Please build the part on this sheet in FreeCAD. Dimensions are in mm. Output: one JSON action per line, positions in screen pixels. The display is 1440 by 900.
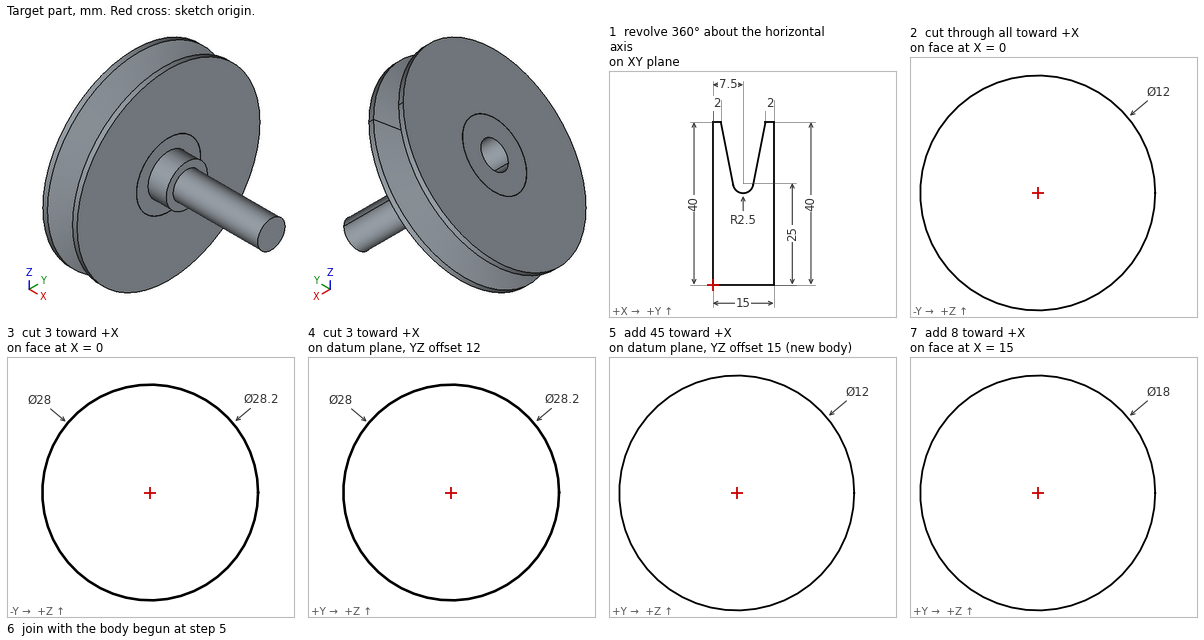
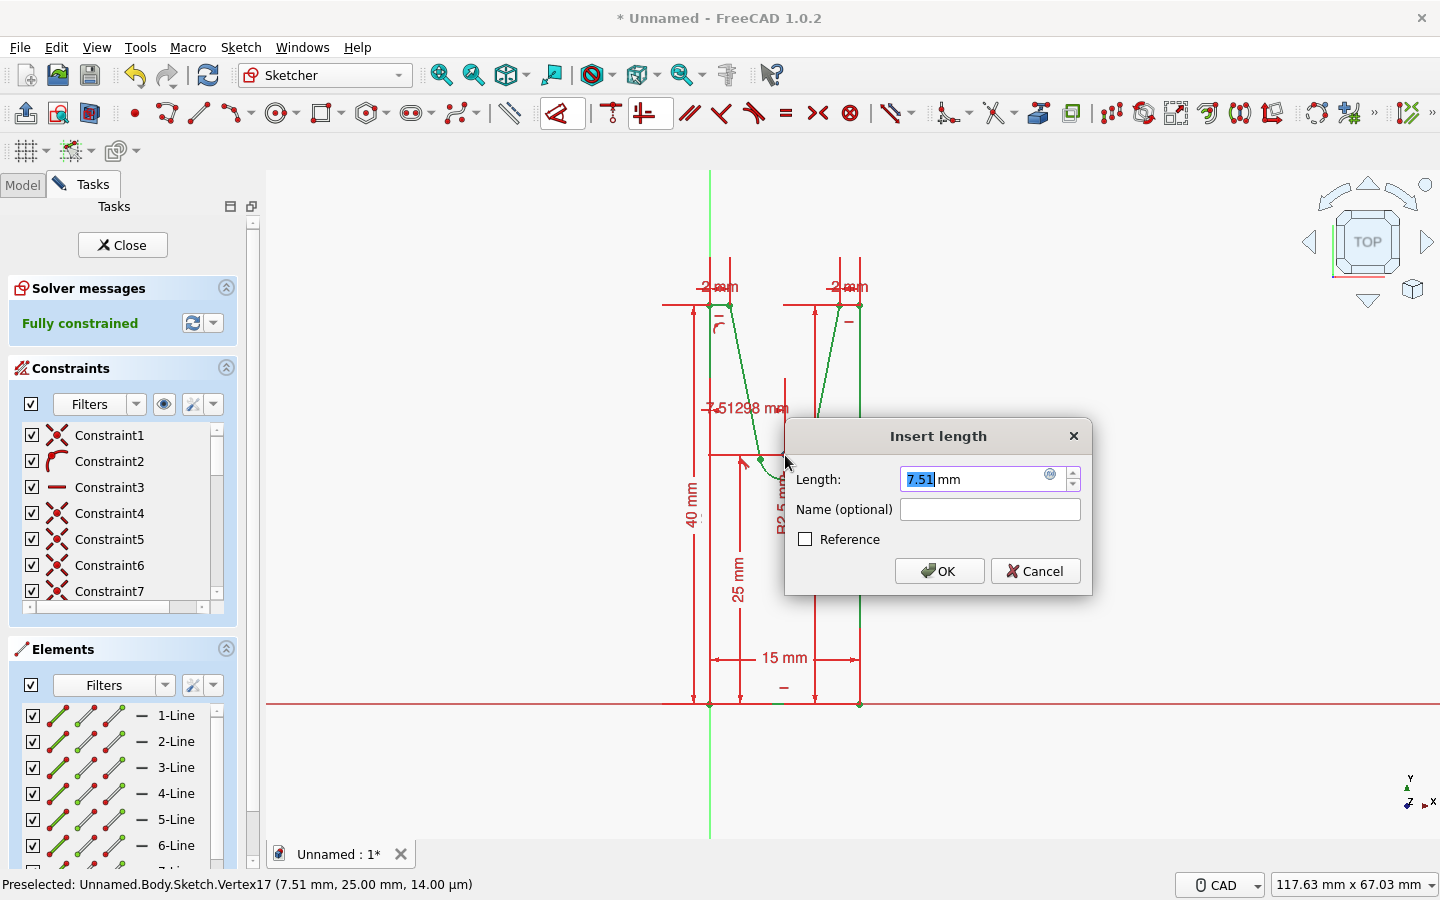
{"action": "type", "text": "7.5"}
{"action": "key", "text": "Return"}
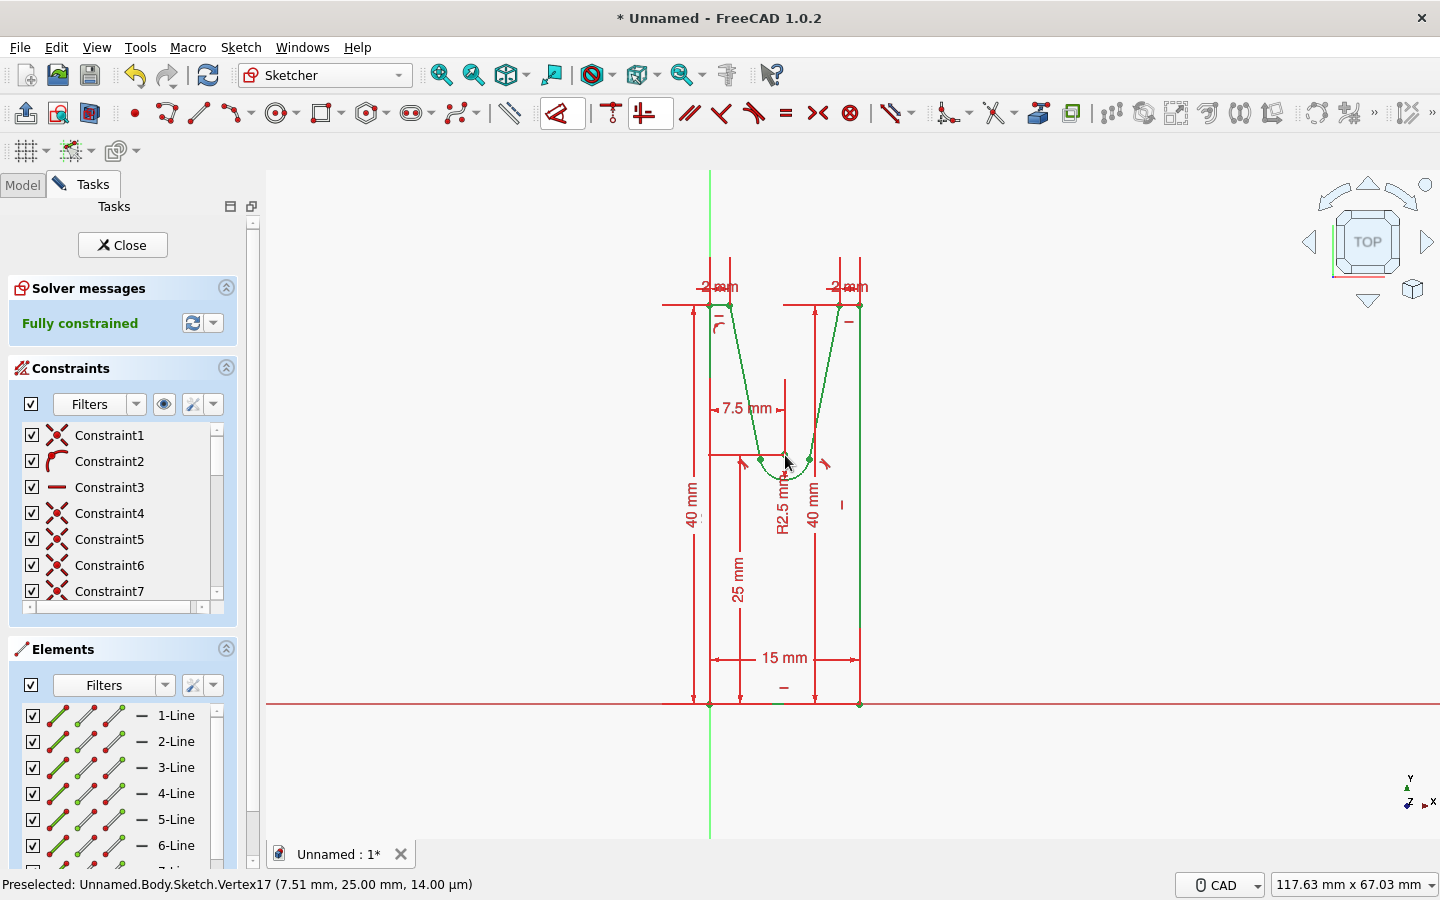
{"action": "left_click", "coordinate": [123, 245]}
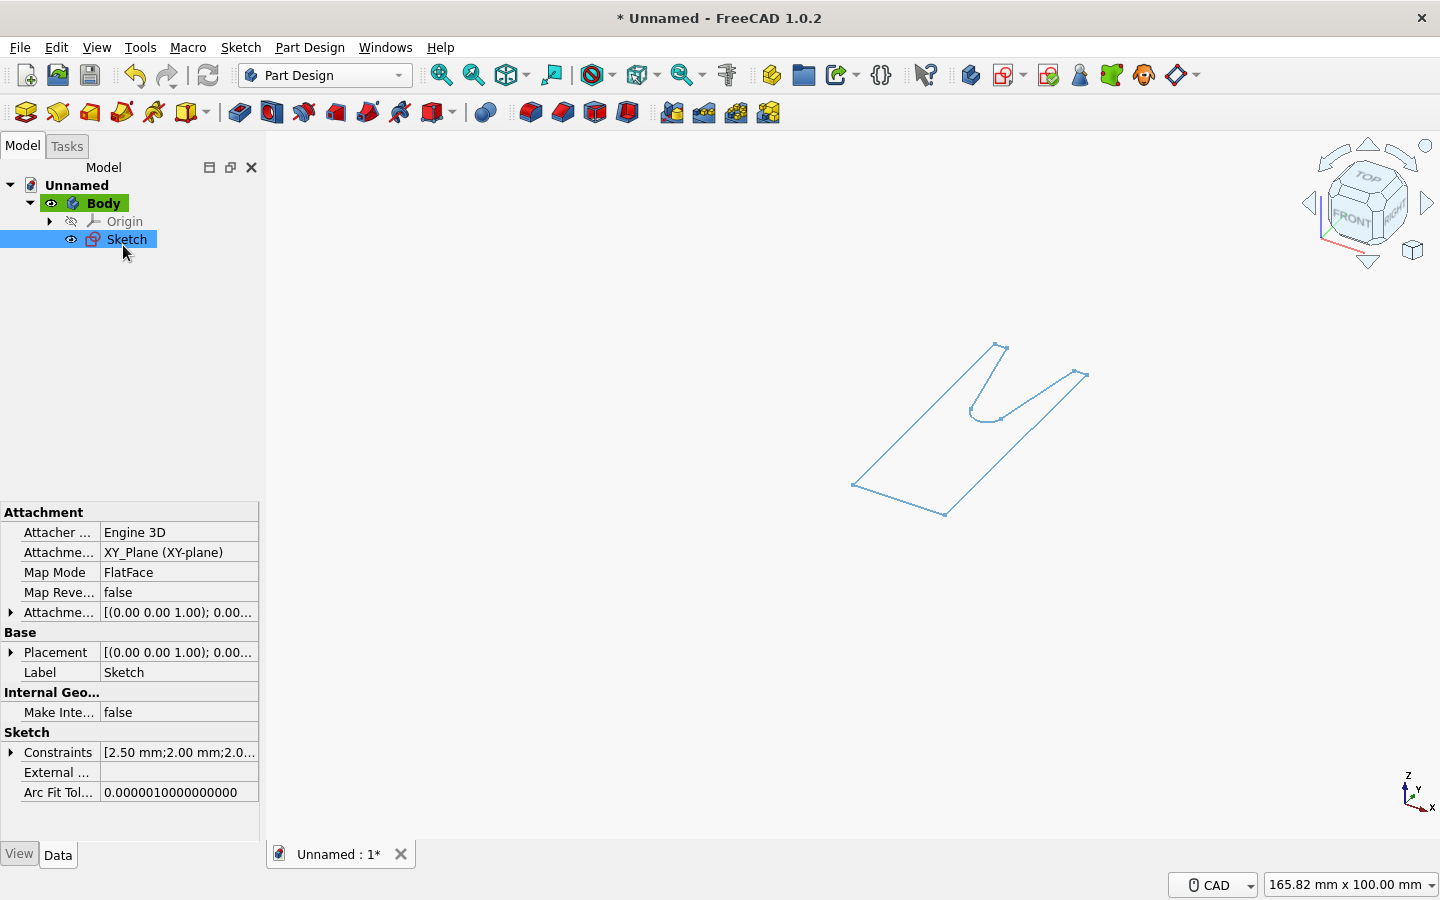
{"action": "left_click", "coordinate": [58, 112]}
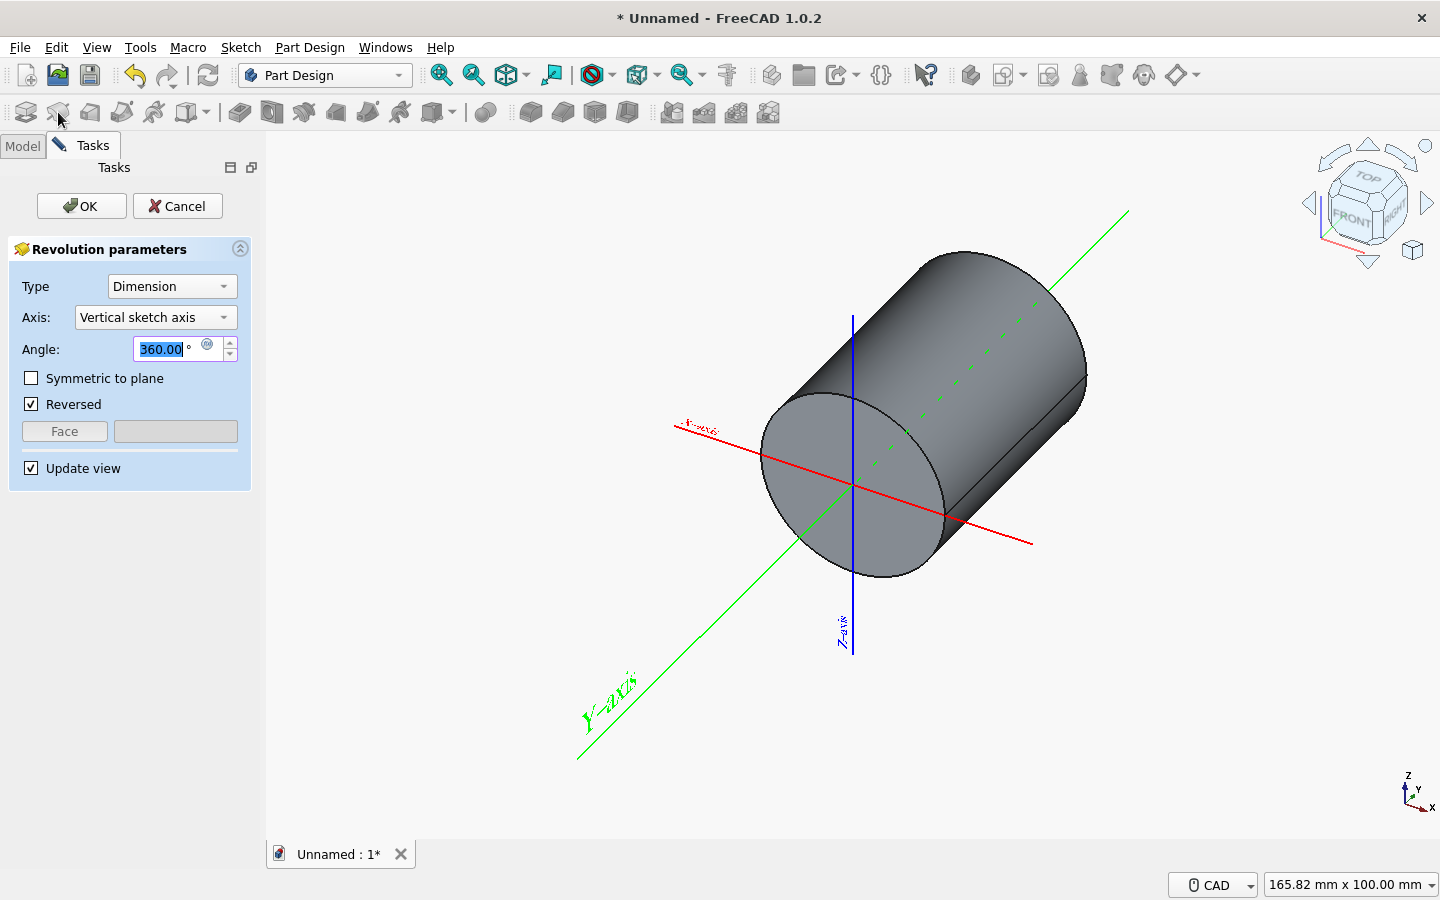
{"action": "left_click", "coordinate": [156, 318]}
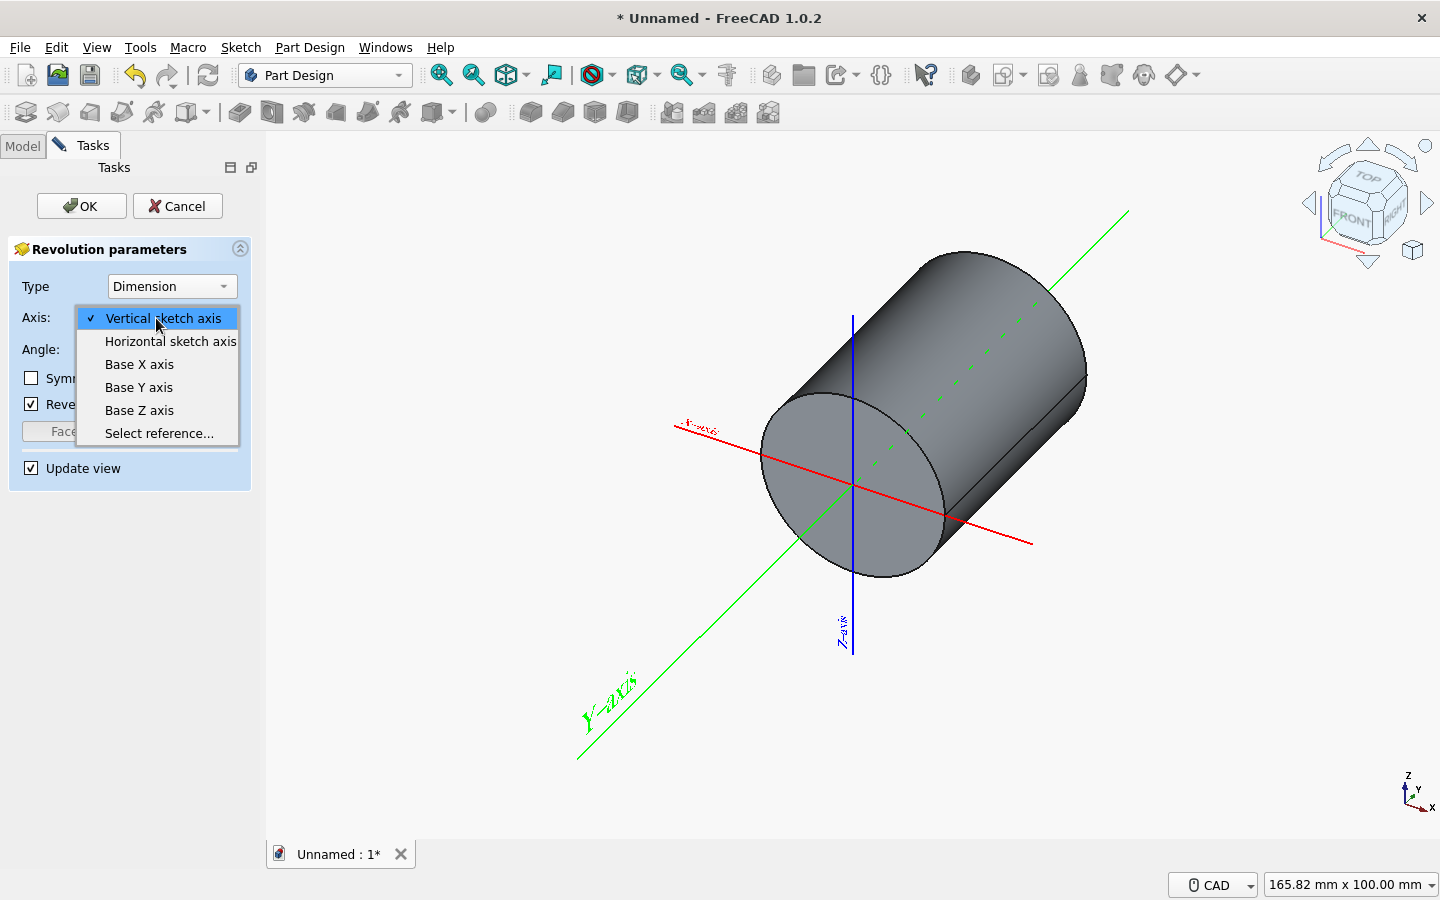
{"action": "left_click", "coordinate": [156, 342]}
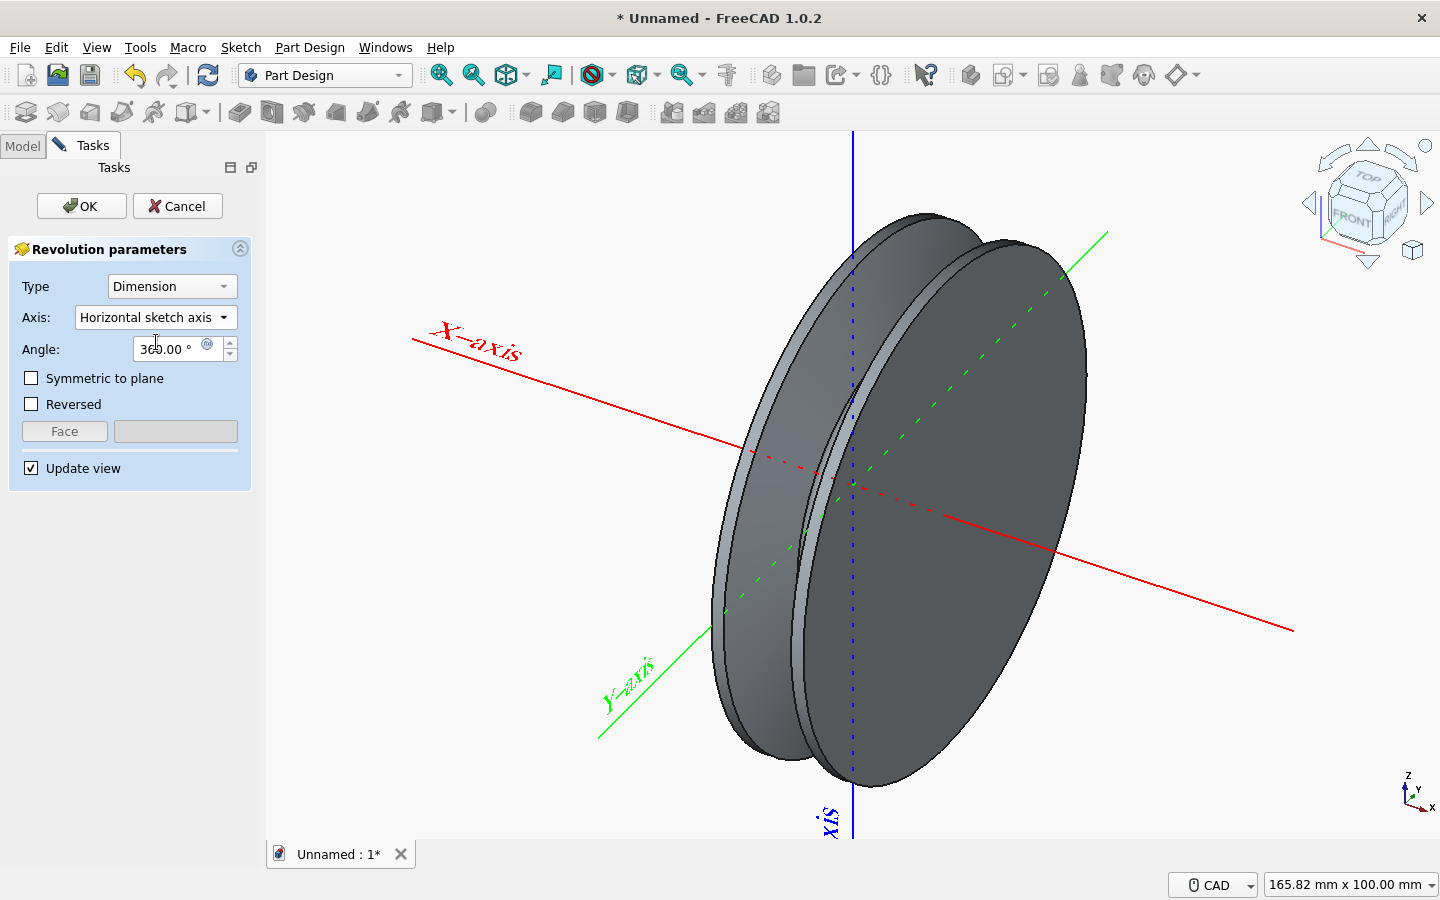
{"action": "left_click", "coordinate": [82, 206]}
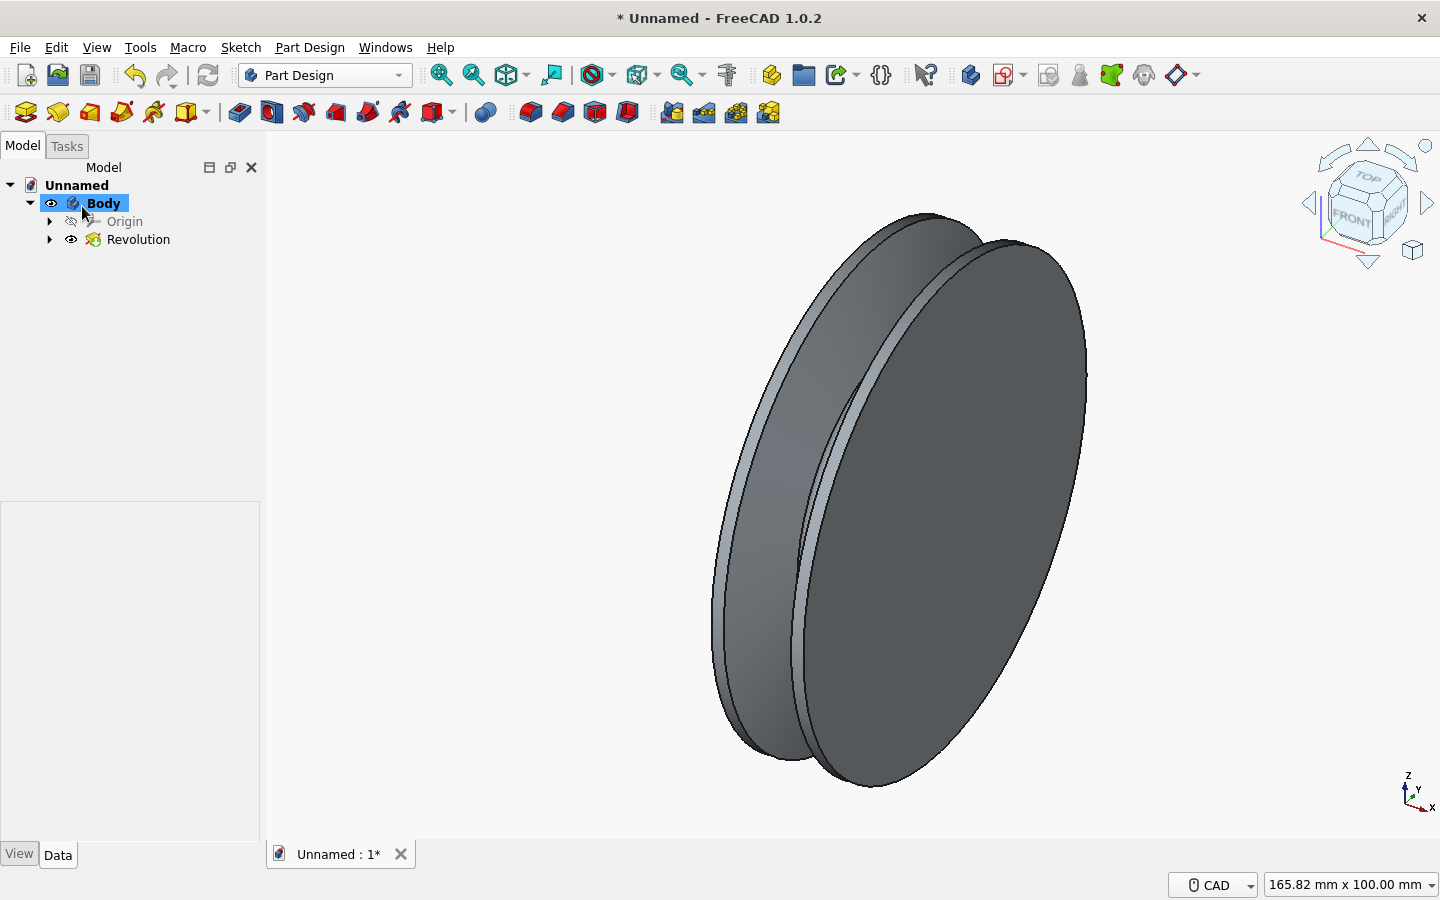
{"action": "left_click", "coordinate": [442, 76]}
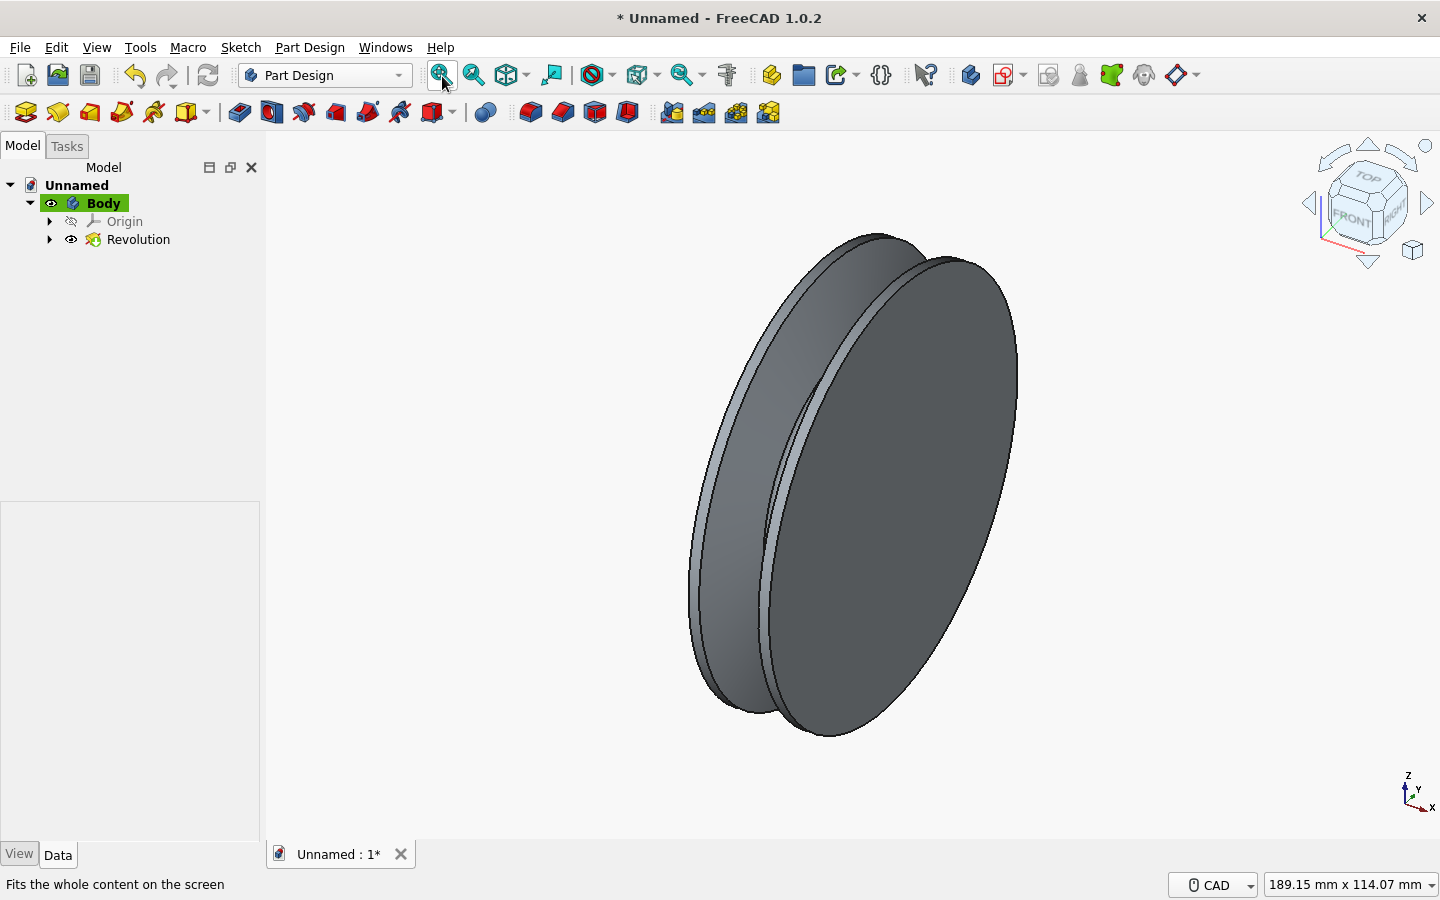
{"action": "key", "text": "6"}